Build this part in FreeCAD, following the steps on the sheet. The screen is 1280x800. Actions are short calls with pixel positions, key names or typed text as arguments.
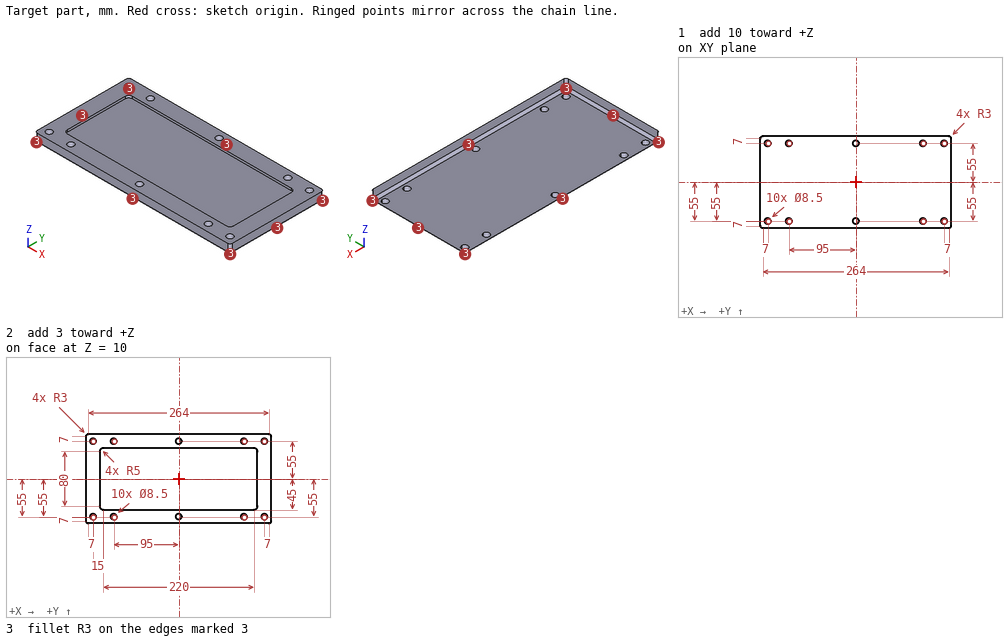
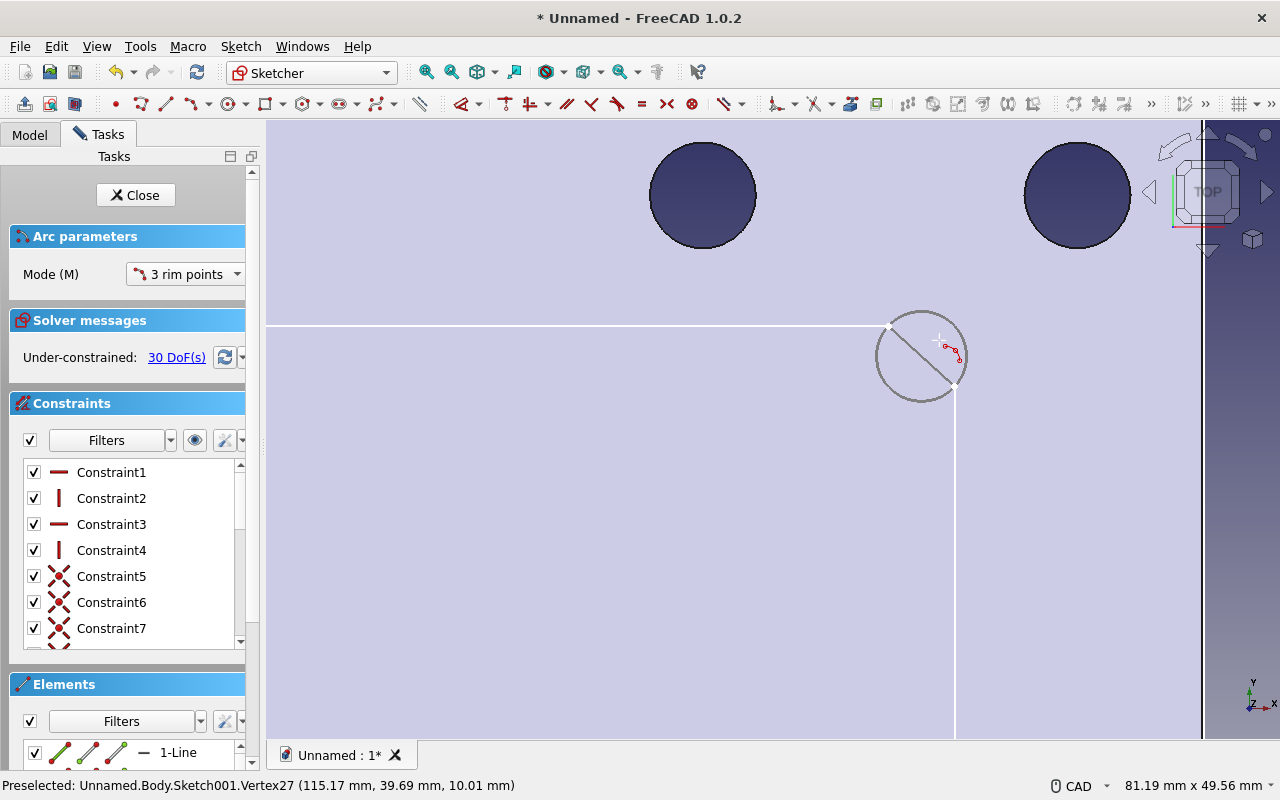
click(934, 339)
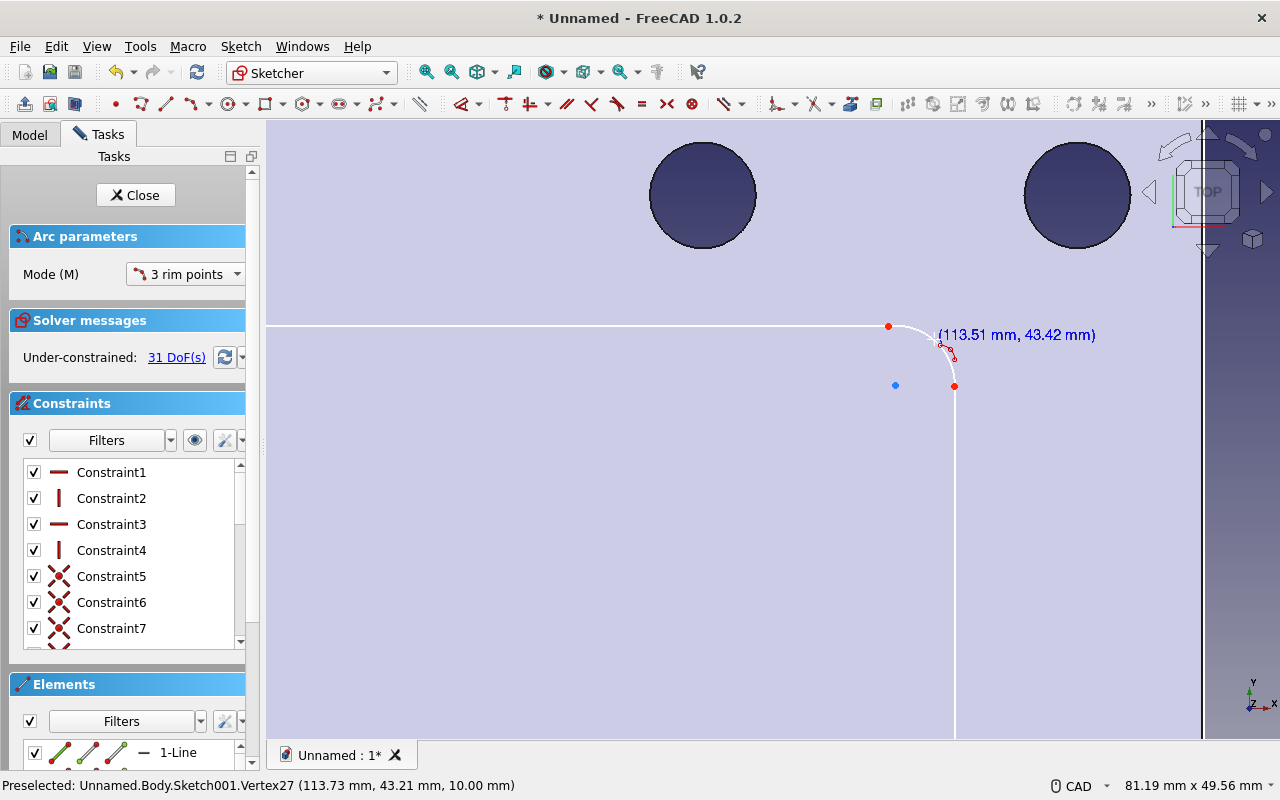
scroll(940, 340, down, 9)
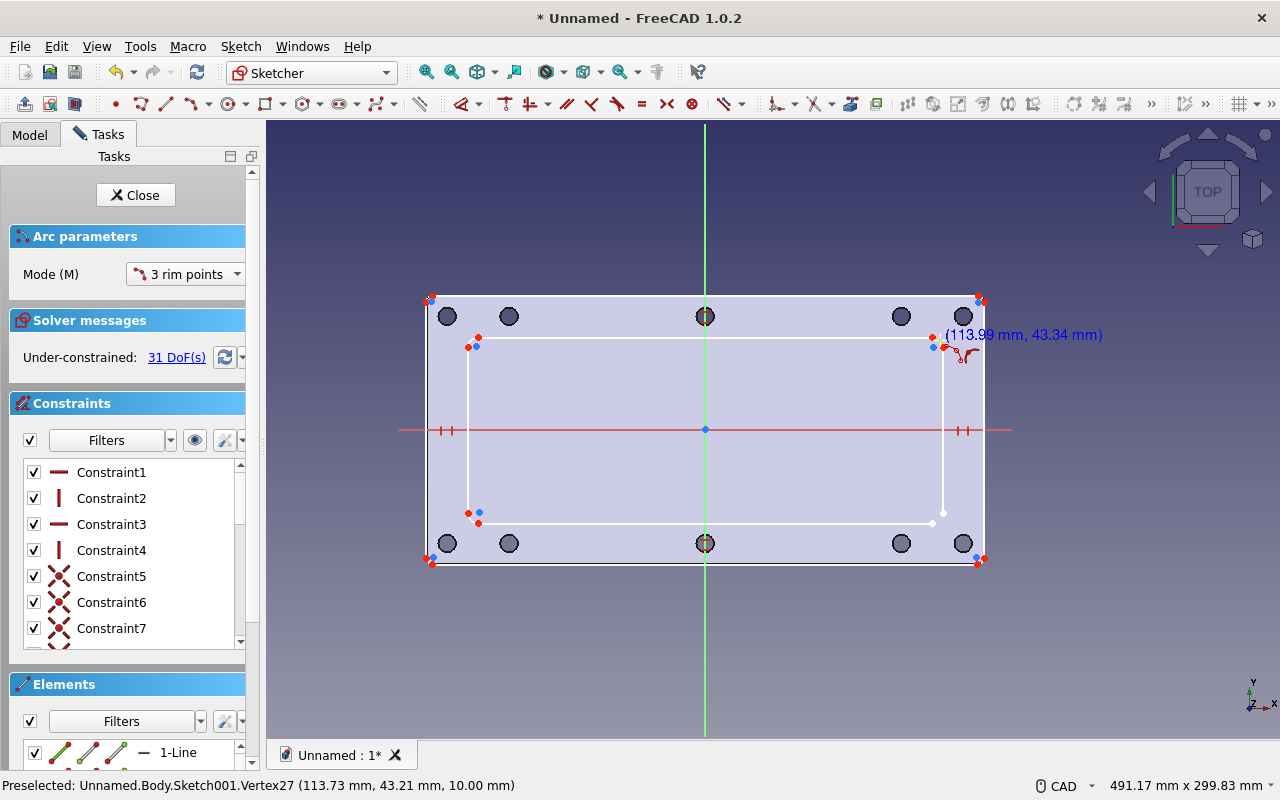
click(943, 514)
click(932, 524)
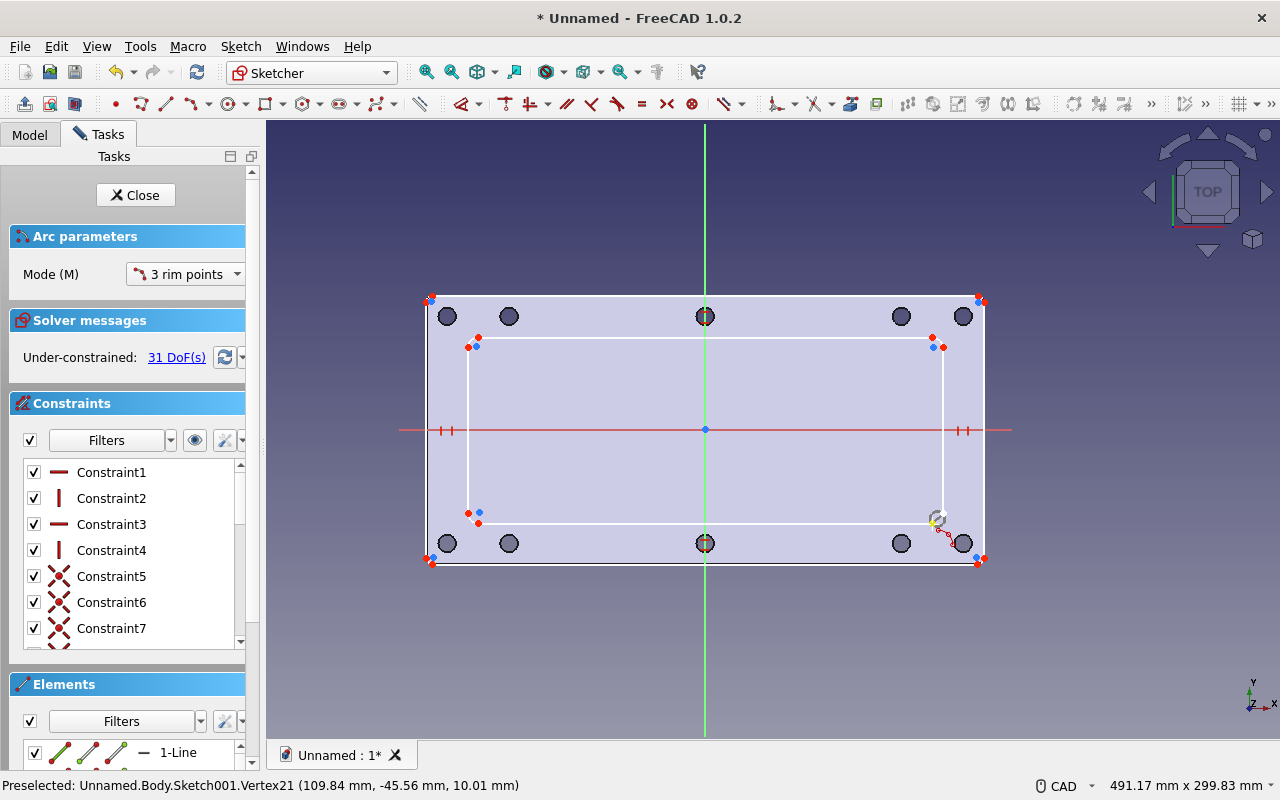
scroll(940, 520, up, 9)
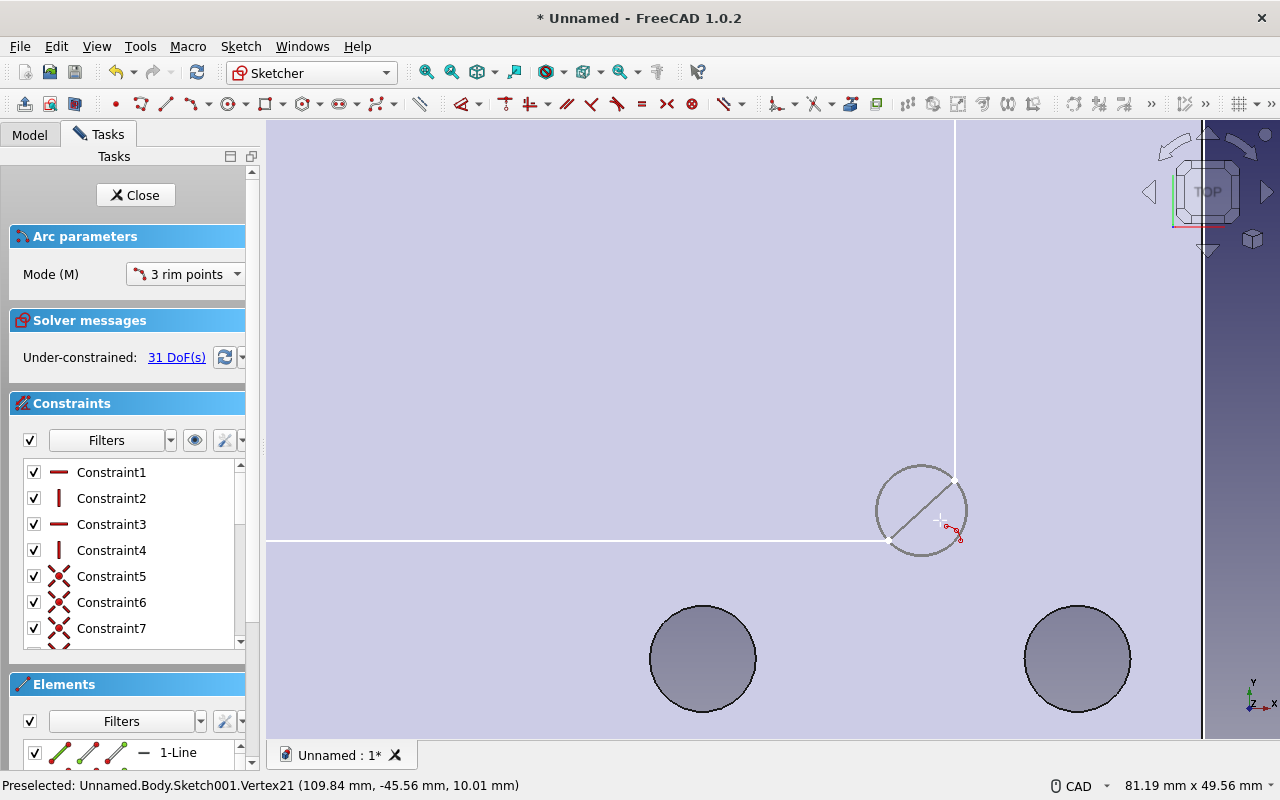
click(934, 516)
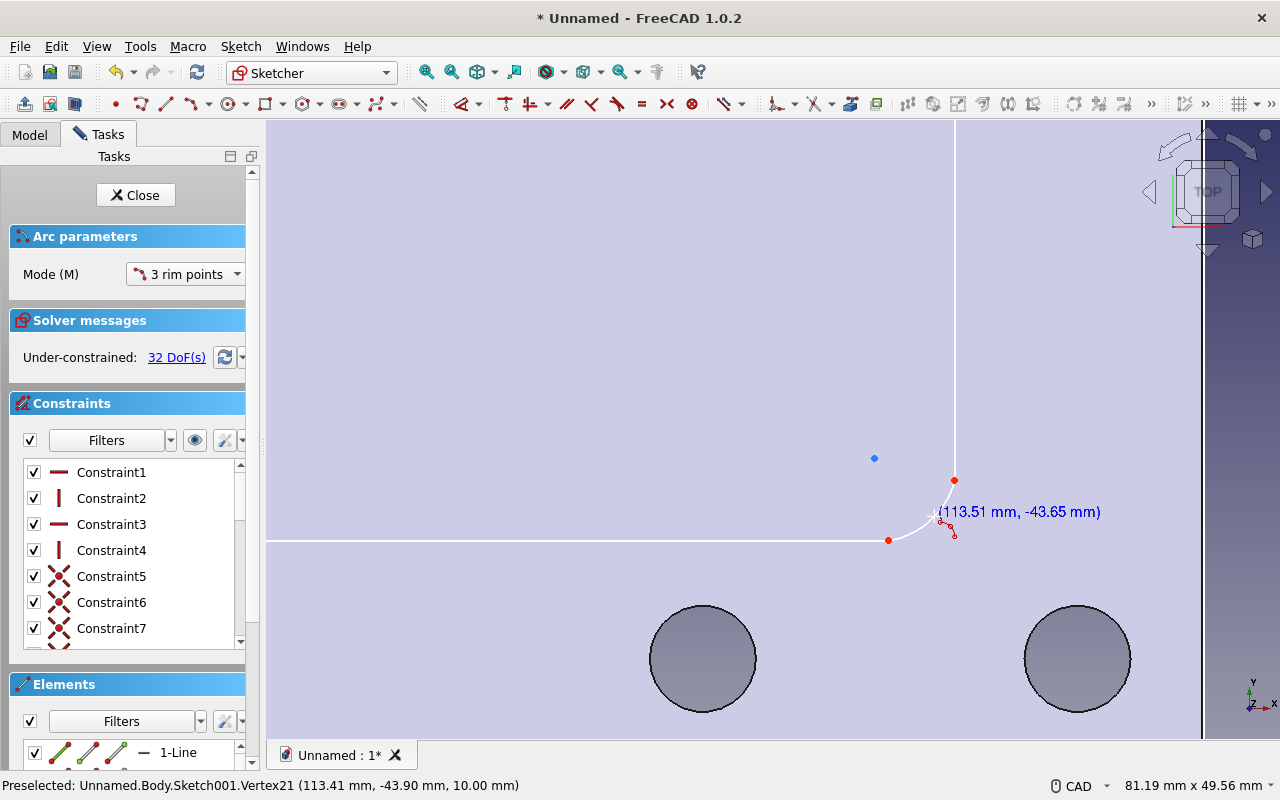
click(228, 104)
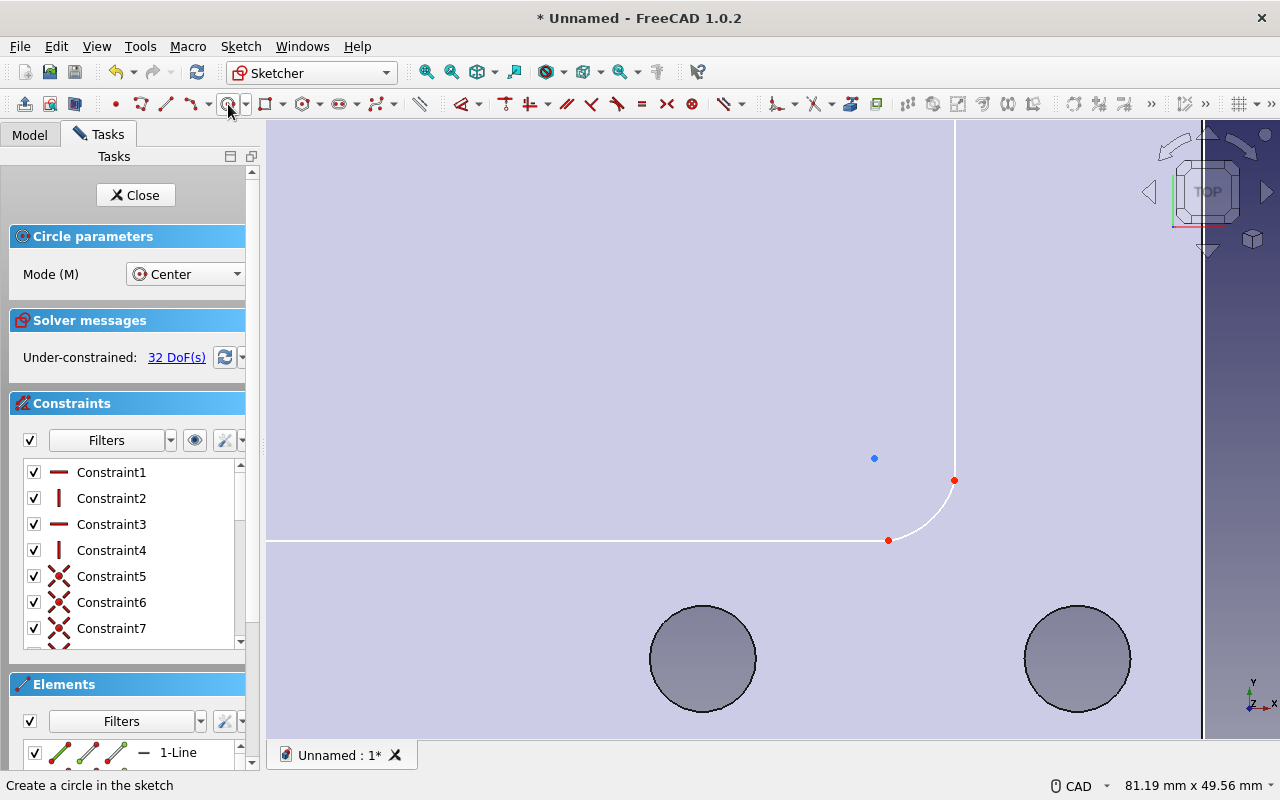
scroll(940, 520, down, 9)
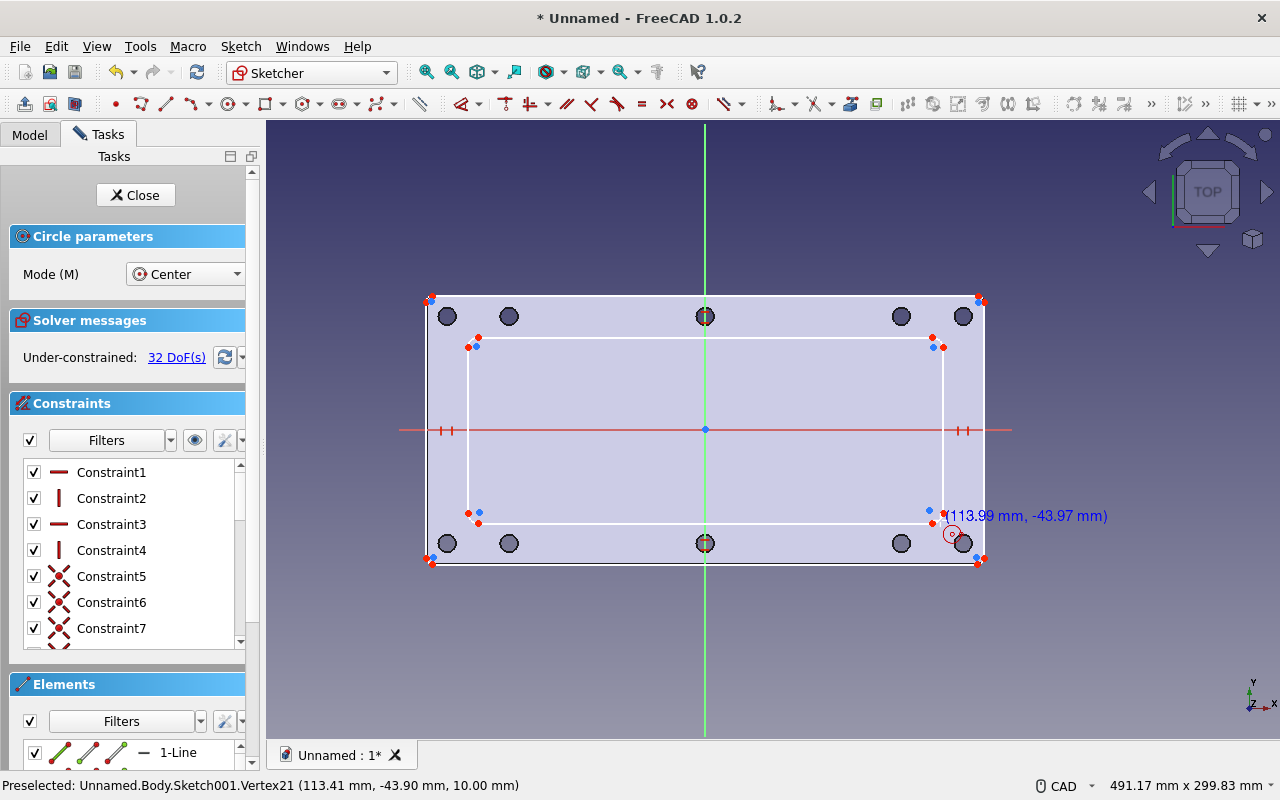
scroll(447, 543, up, 5)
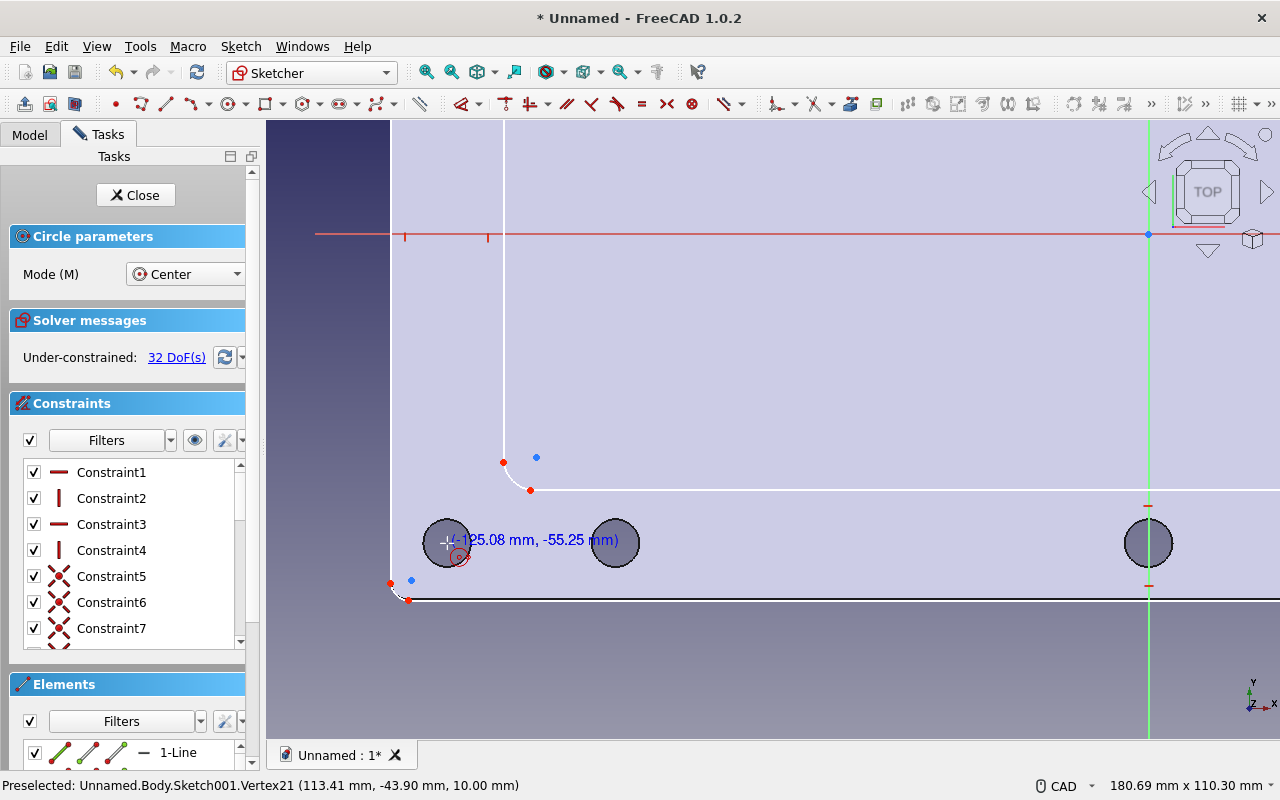
click(447, 543)
move(464, 526)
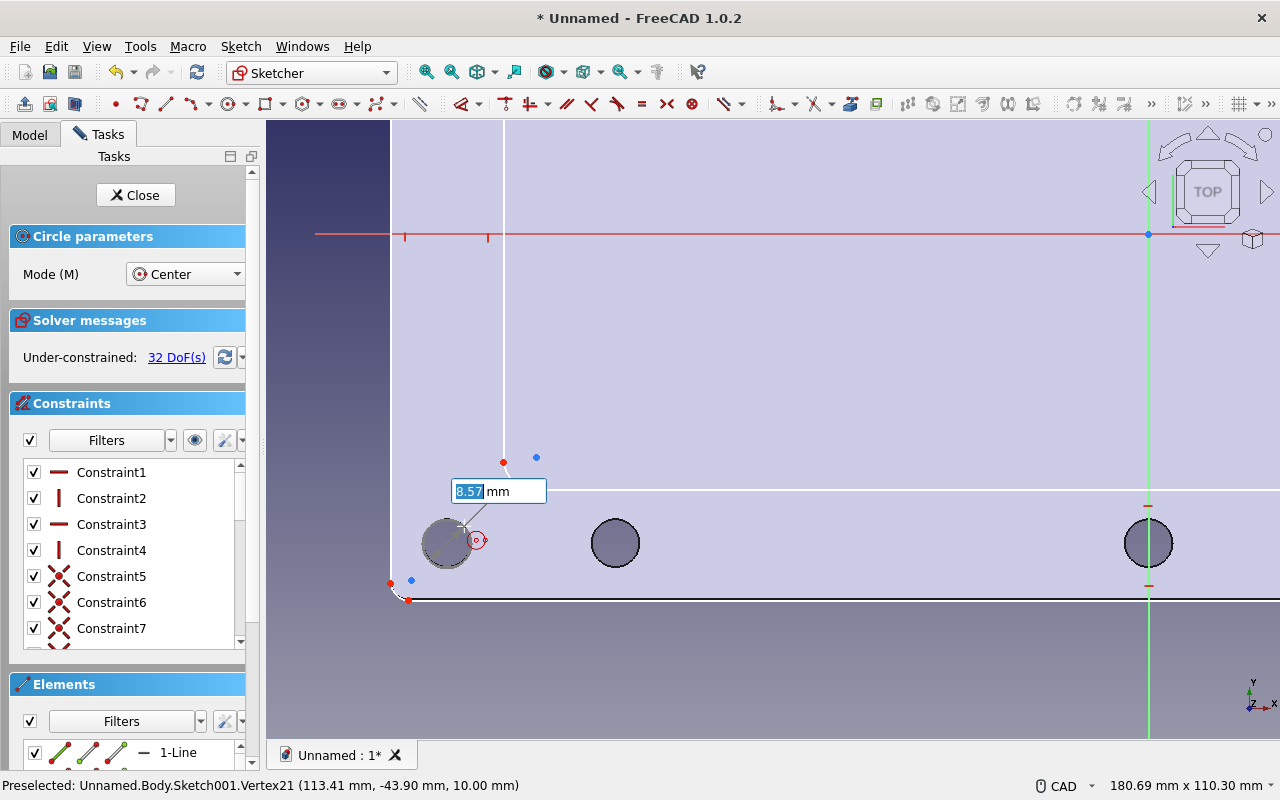
text(8.5)
key(Return)